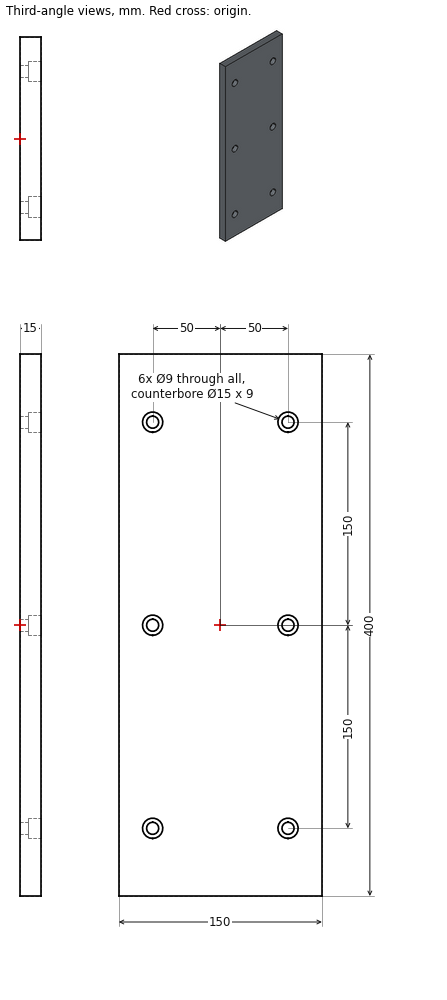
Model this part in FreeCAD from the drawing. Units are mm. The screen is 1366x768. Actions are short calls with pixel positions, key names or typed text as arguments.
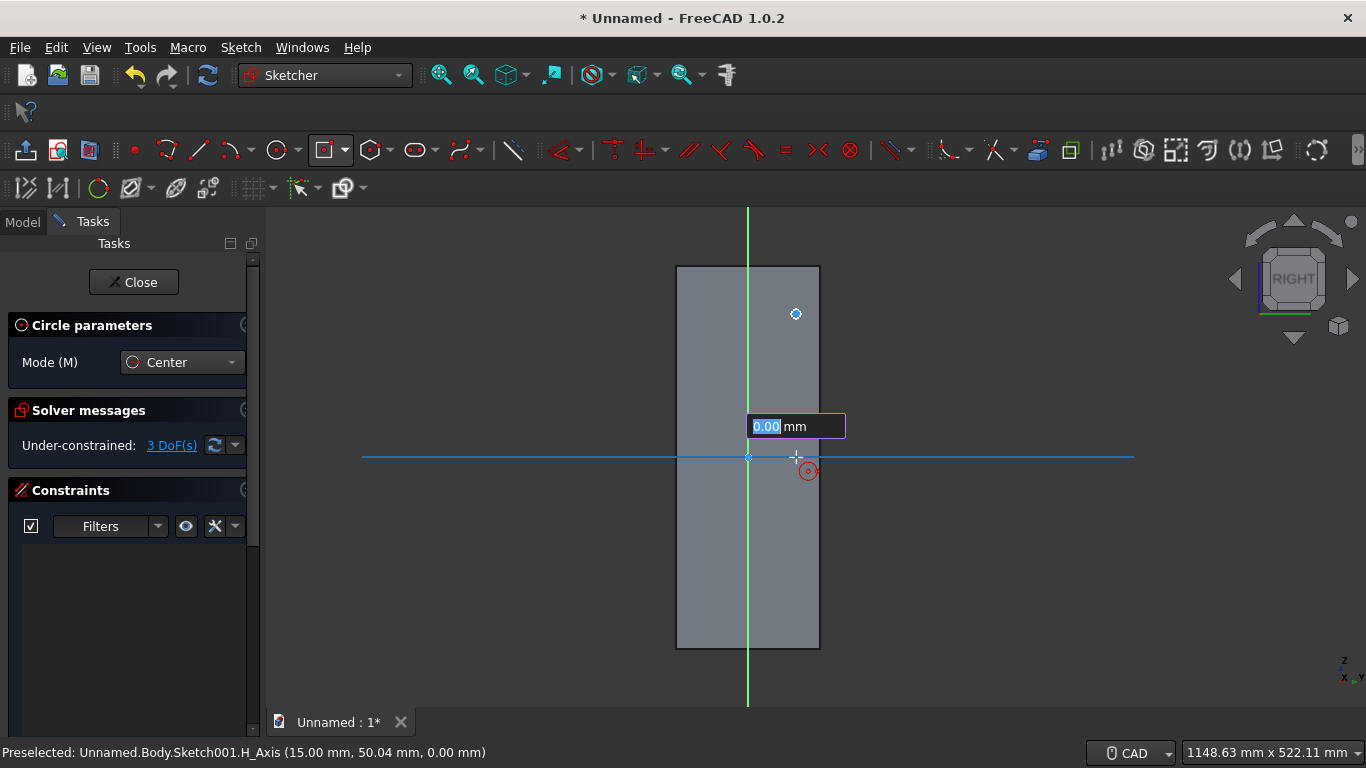
scroll(794, 461, up, 7)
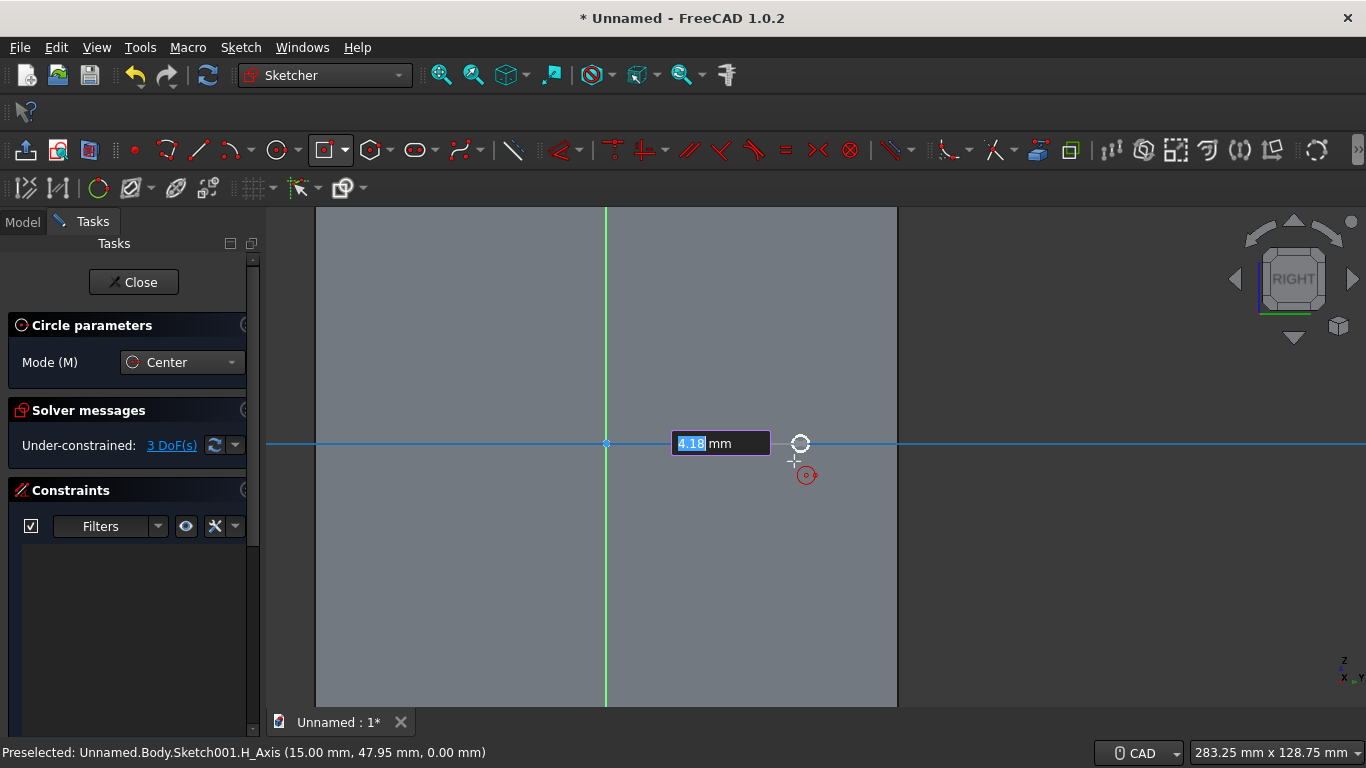
click(795, 460)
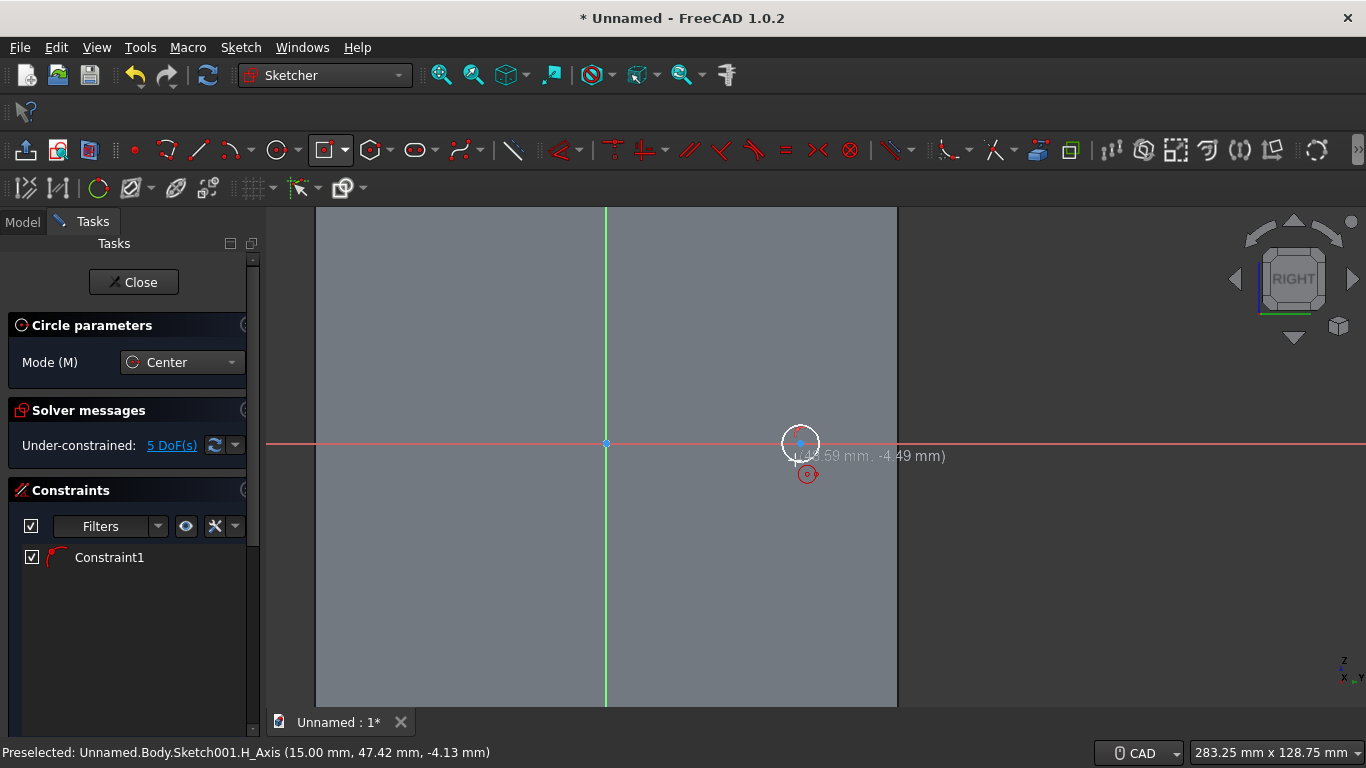
scroll(794, 461, down, 7)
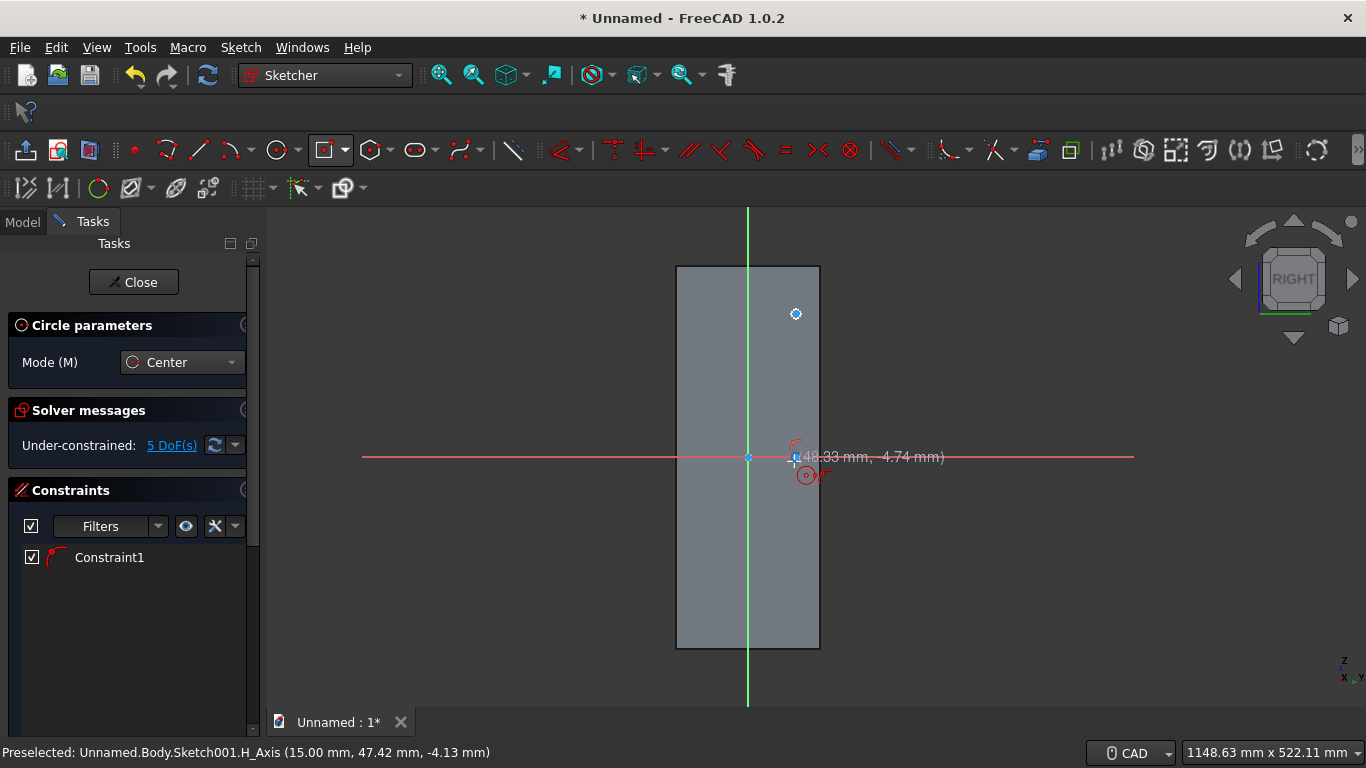
scroll(796, 601, up, 9)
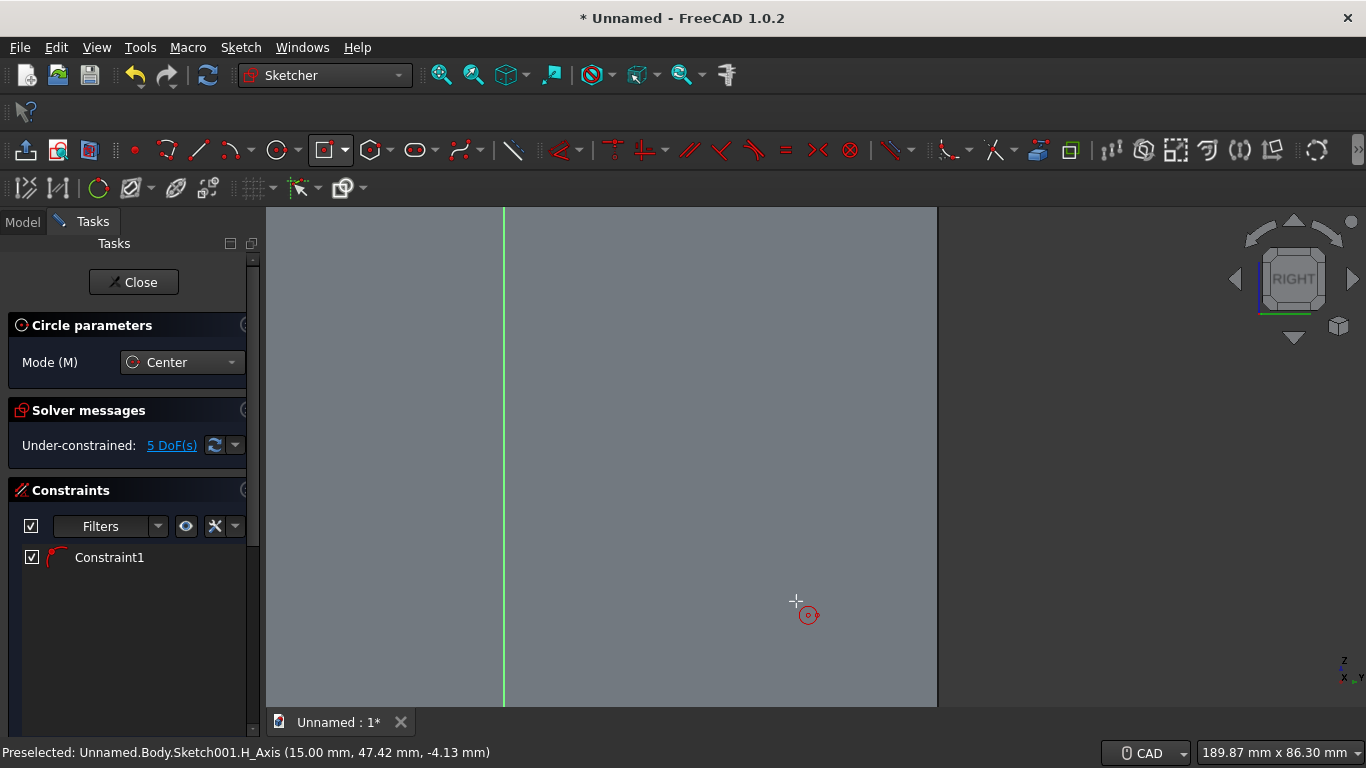
scroll(796, 602, down, 9)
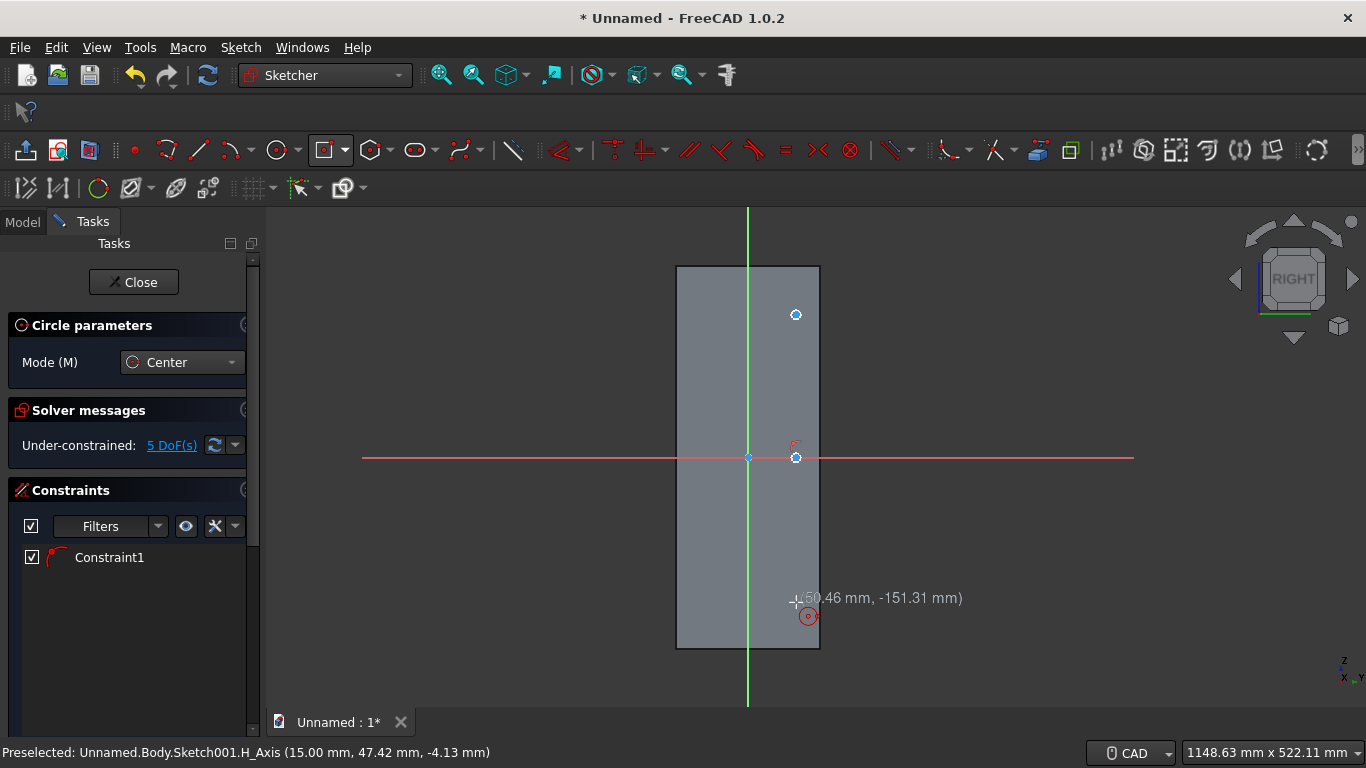
click(796, 602)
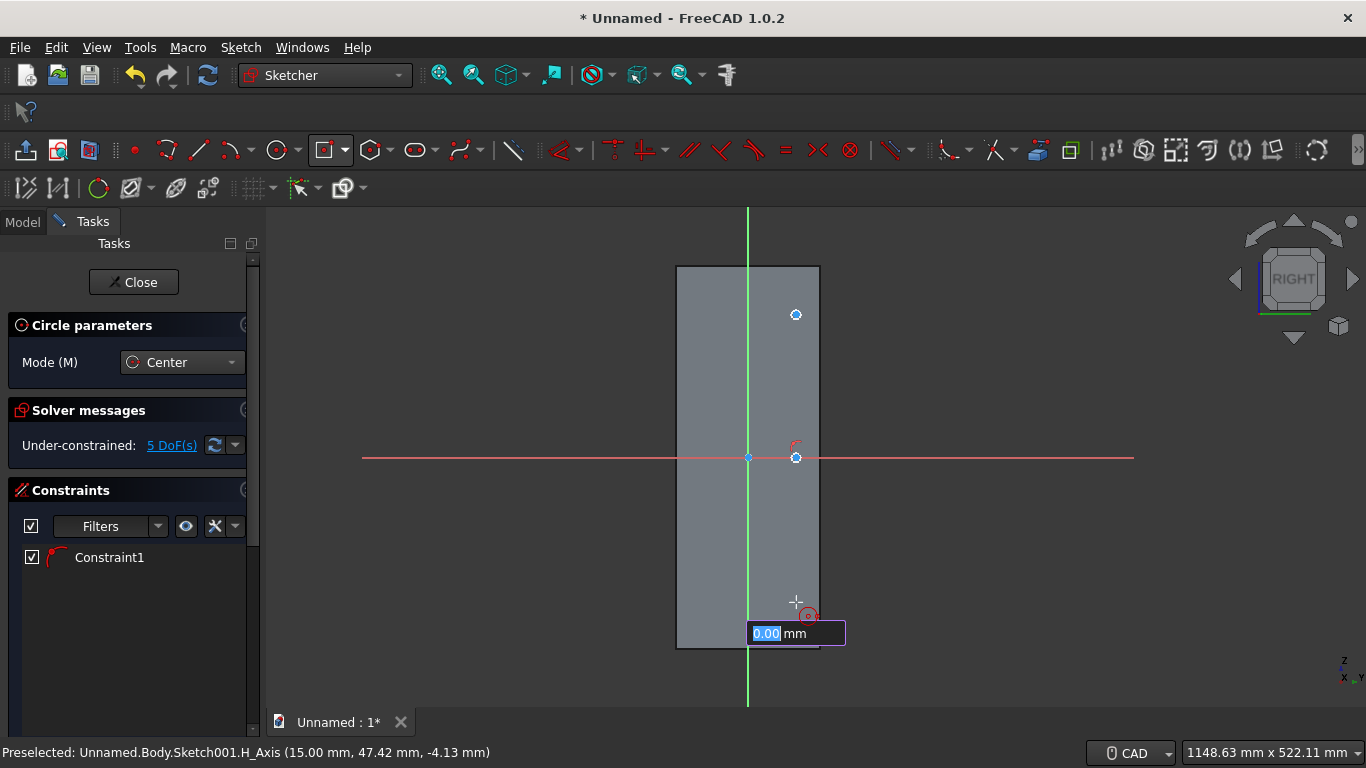
scroll(799, 599, up, 7)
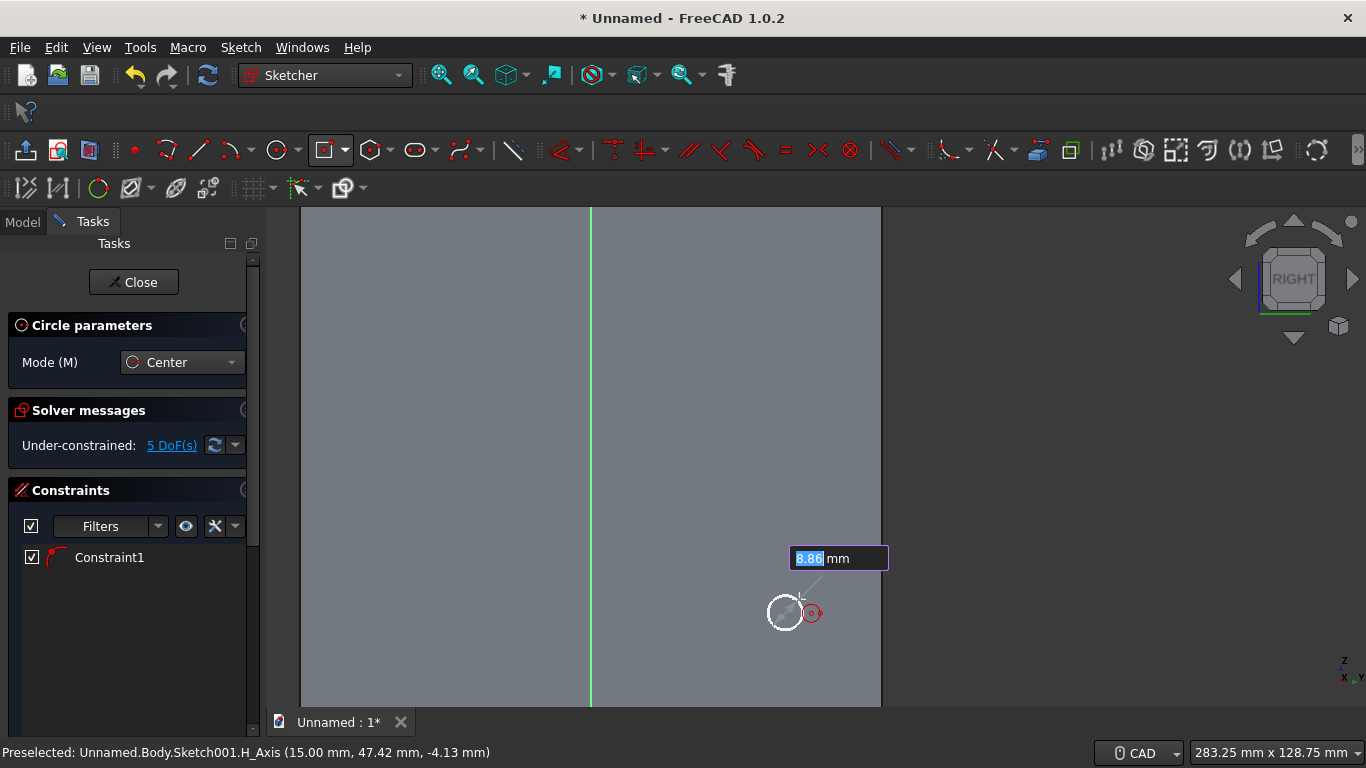
click(798, 595)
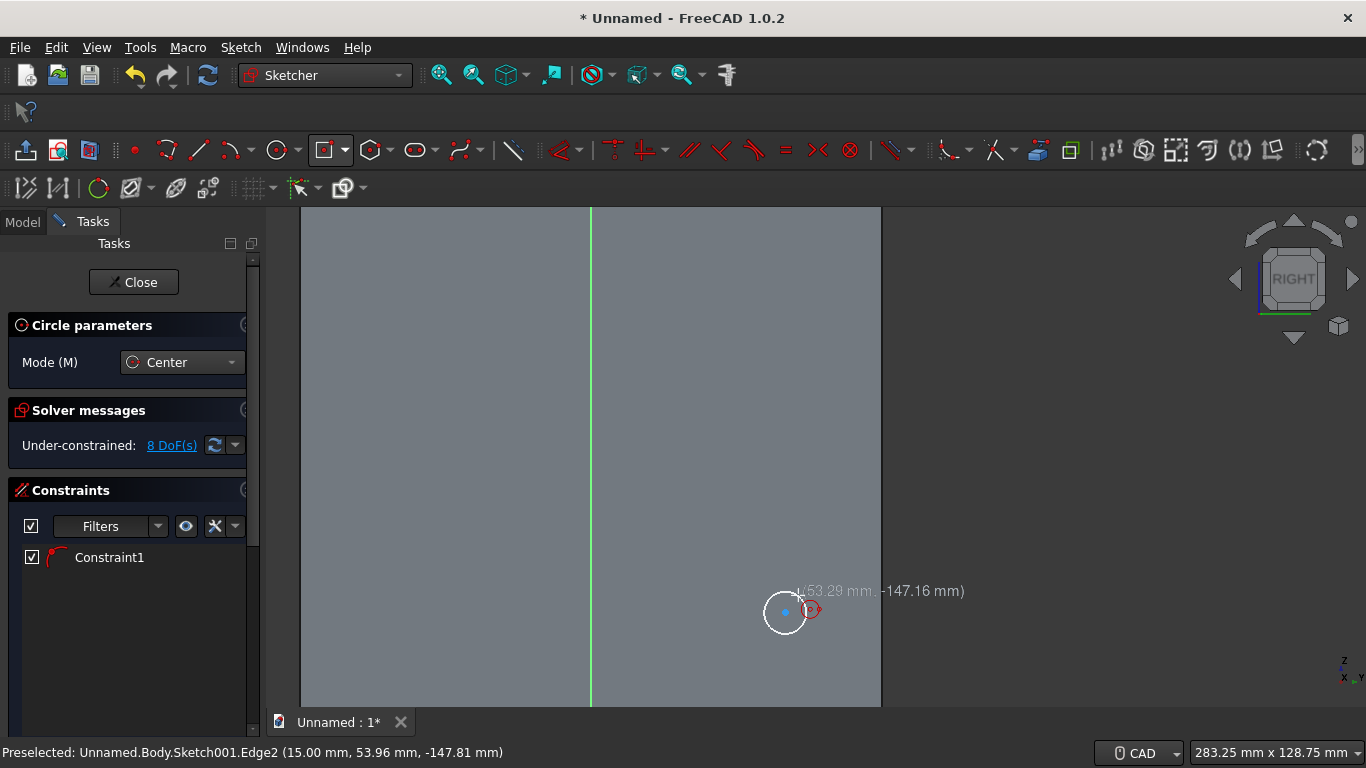
scroll(799, 599, down, 7)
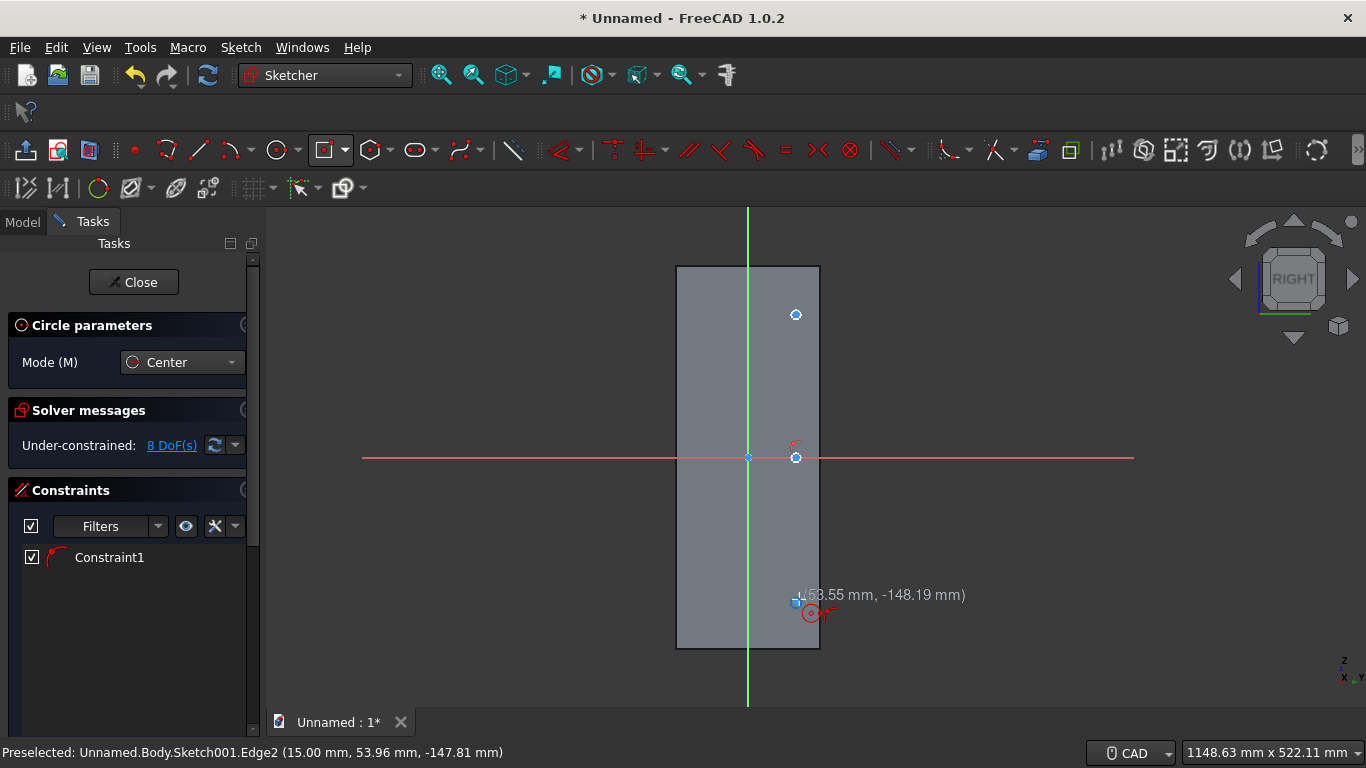
scroll(700, 314, up, 9)